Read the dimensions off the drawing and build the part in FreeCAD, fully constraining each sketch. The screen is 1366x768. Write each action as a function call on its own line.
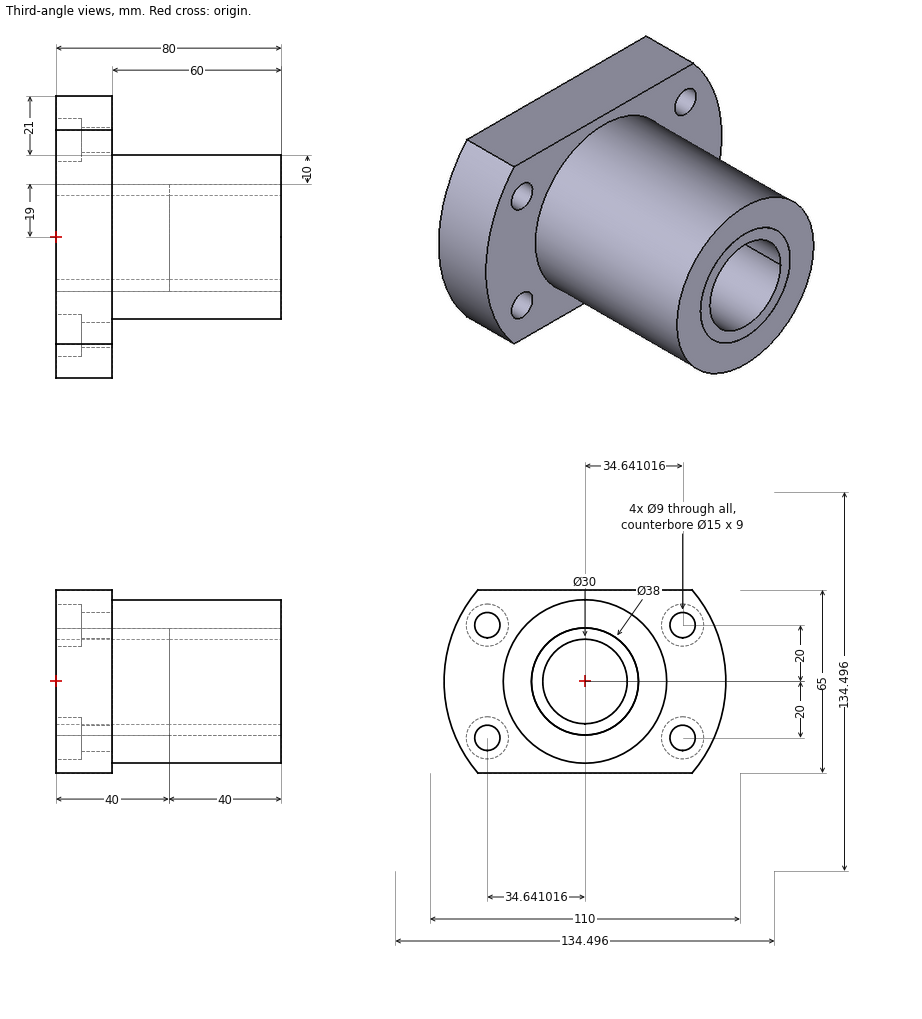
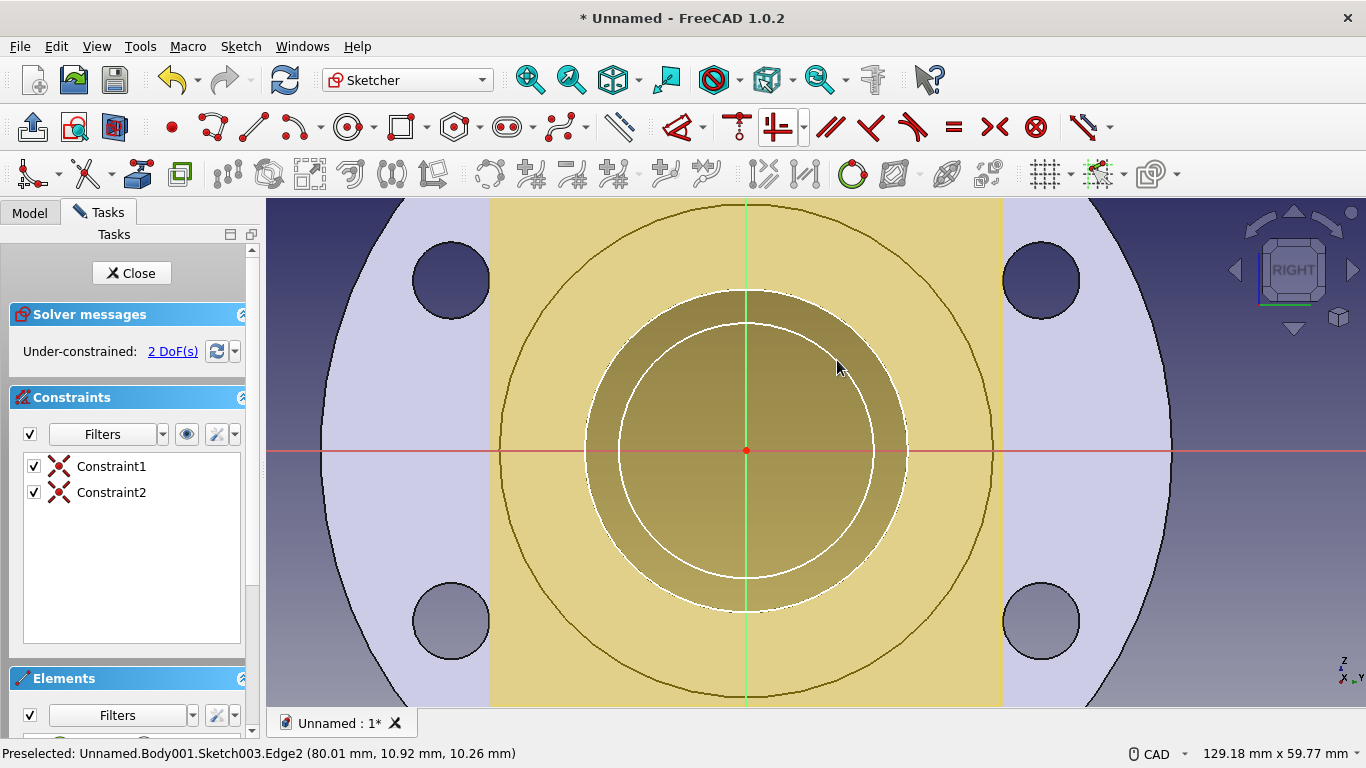
key(d)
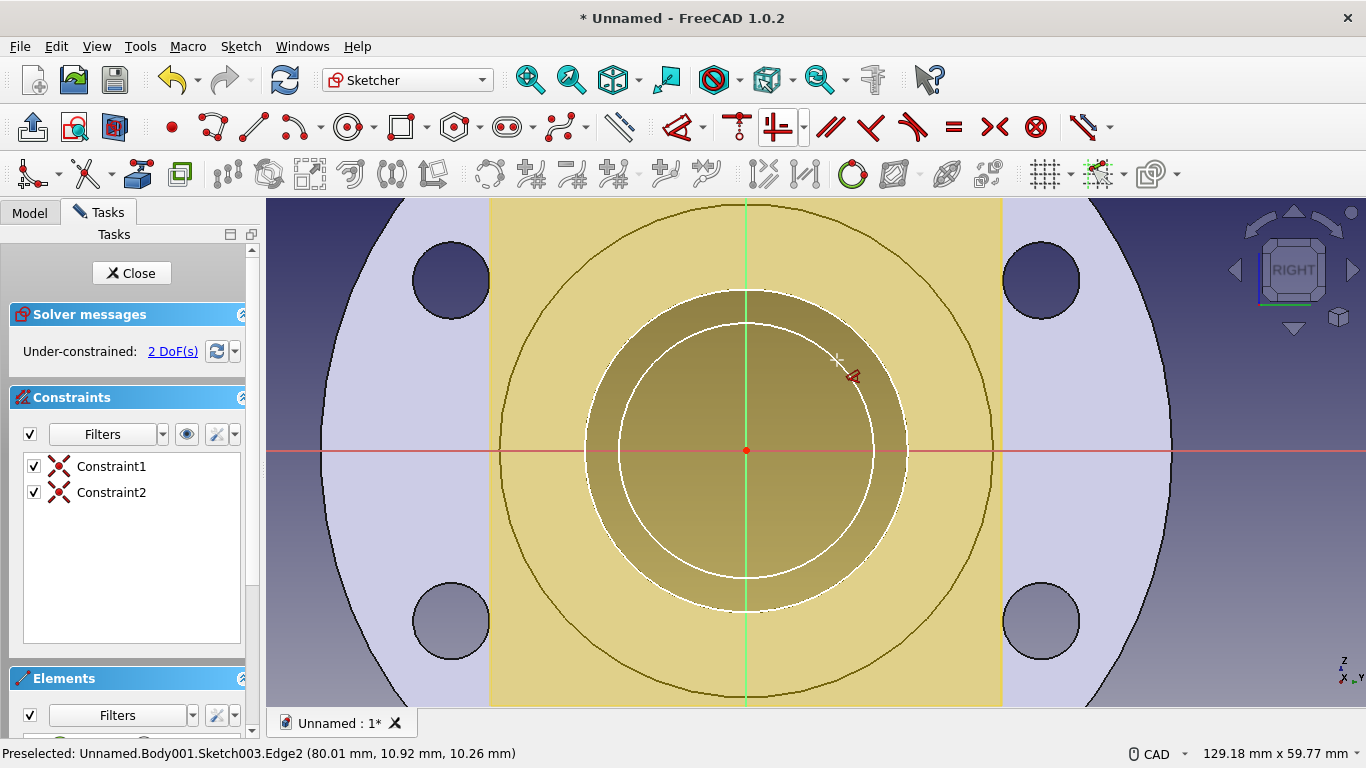
click(860, 336)
click(883, 313)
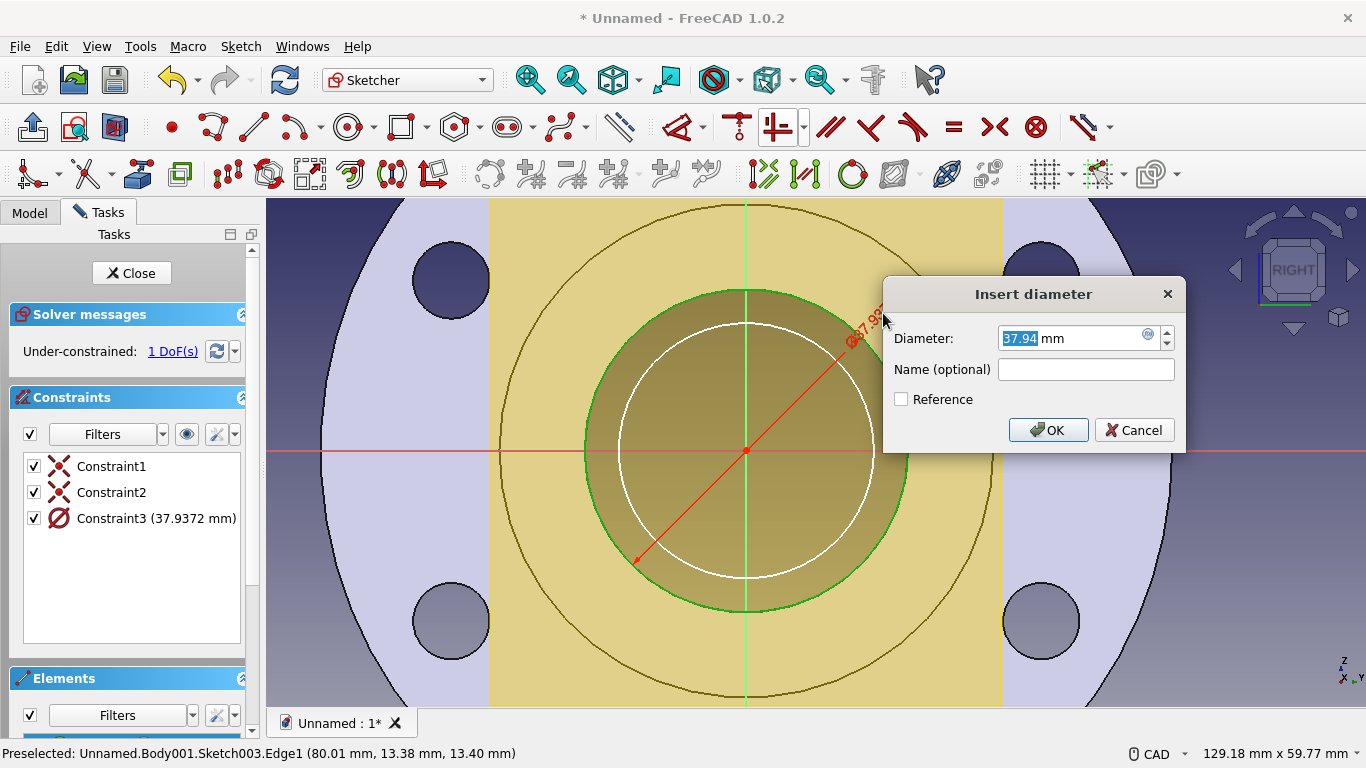
text(38)
key(Return)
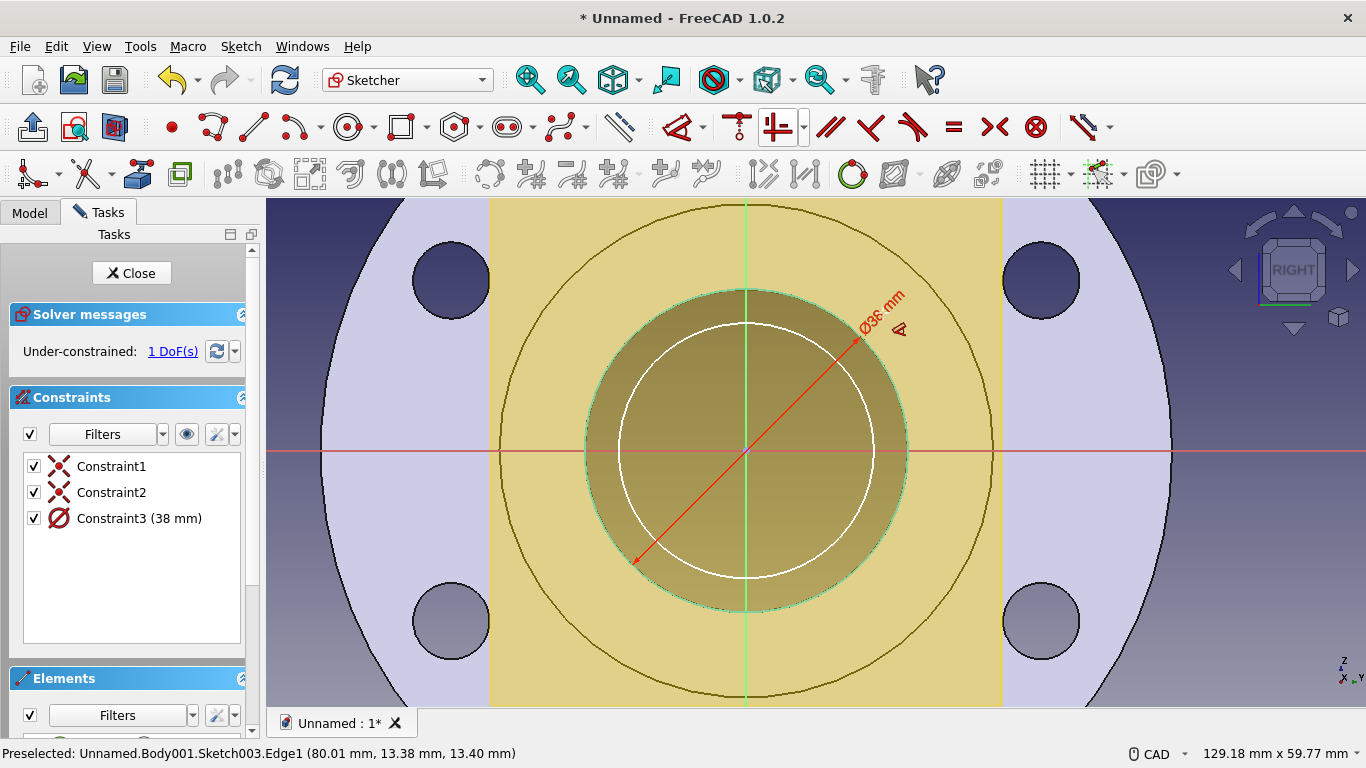
click(836, 360)
click(921, 398)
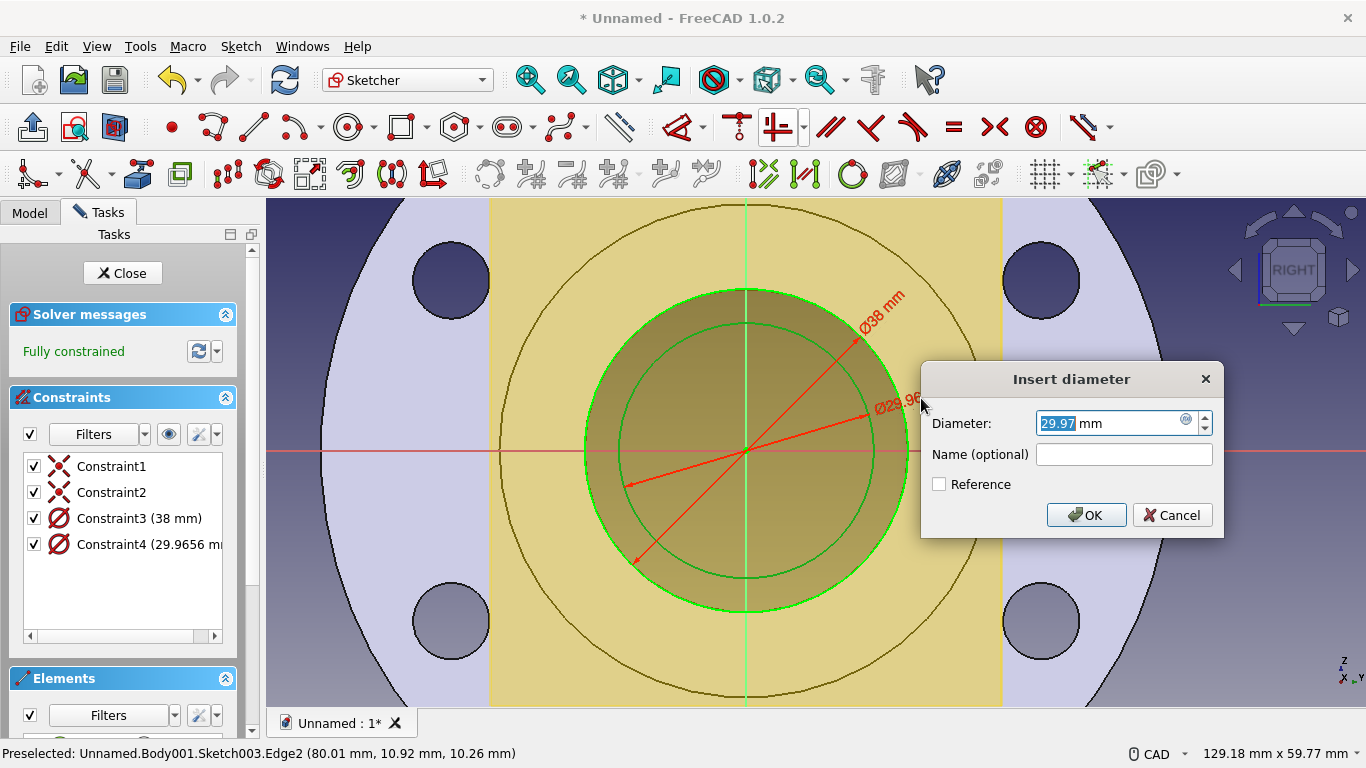
text(30)
key(Return)
key(Escape)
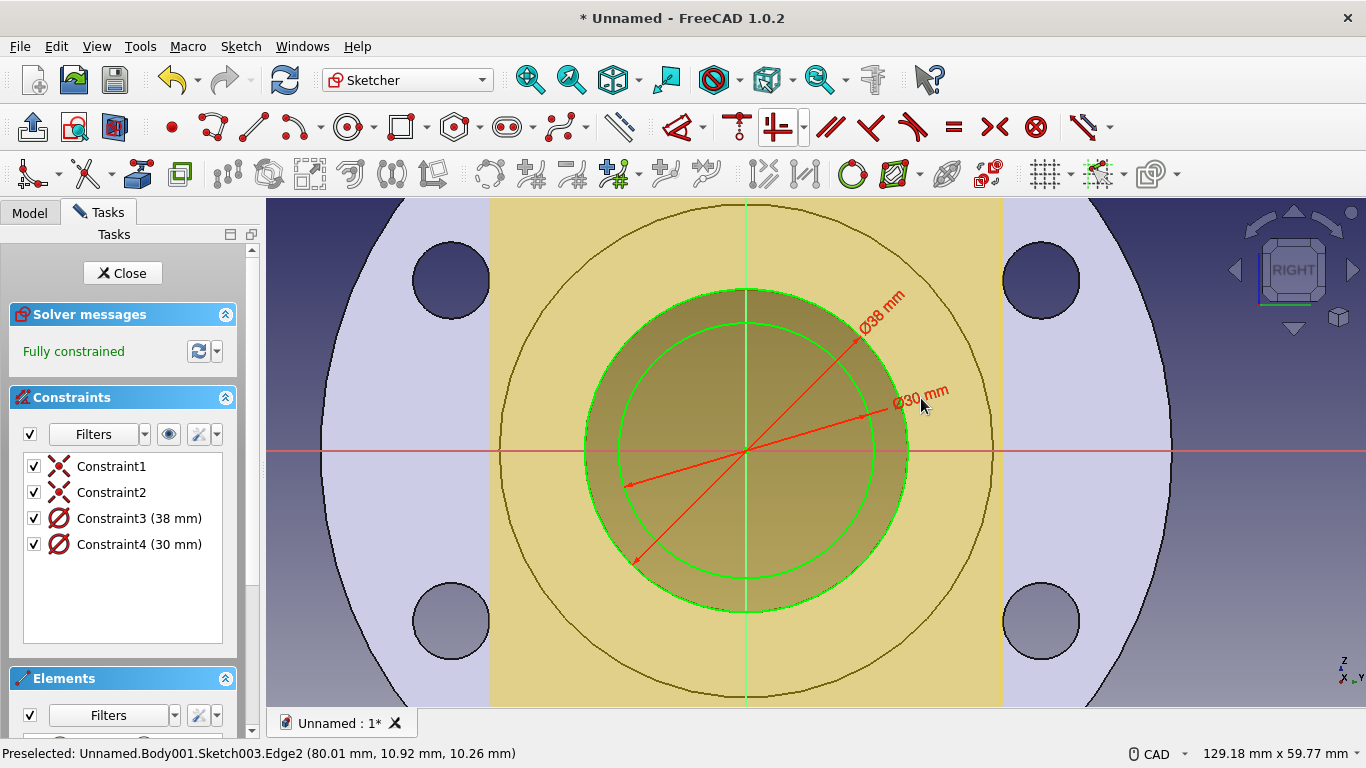
click(123, 273)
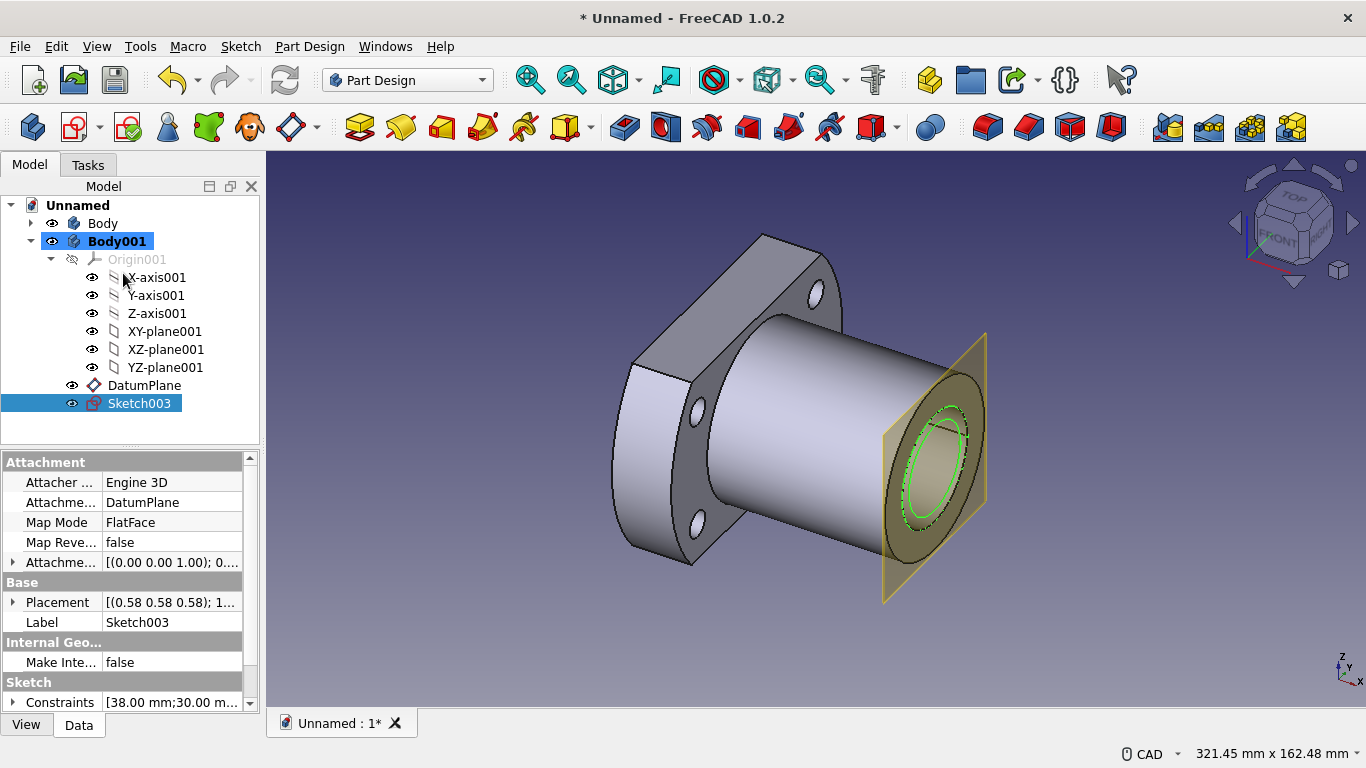
click(360, 128)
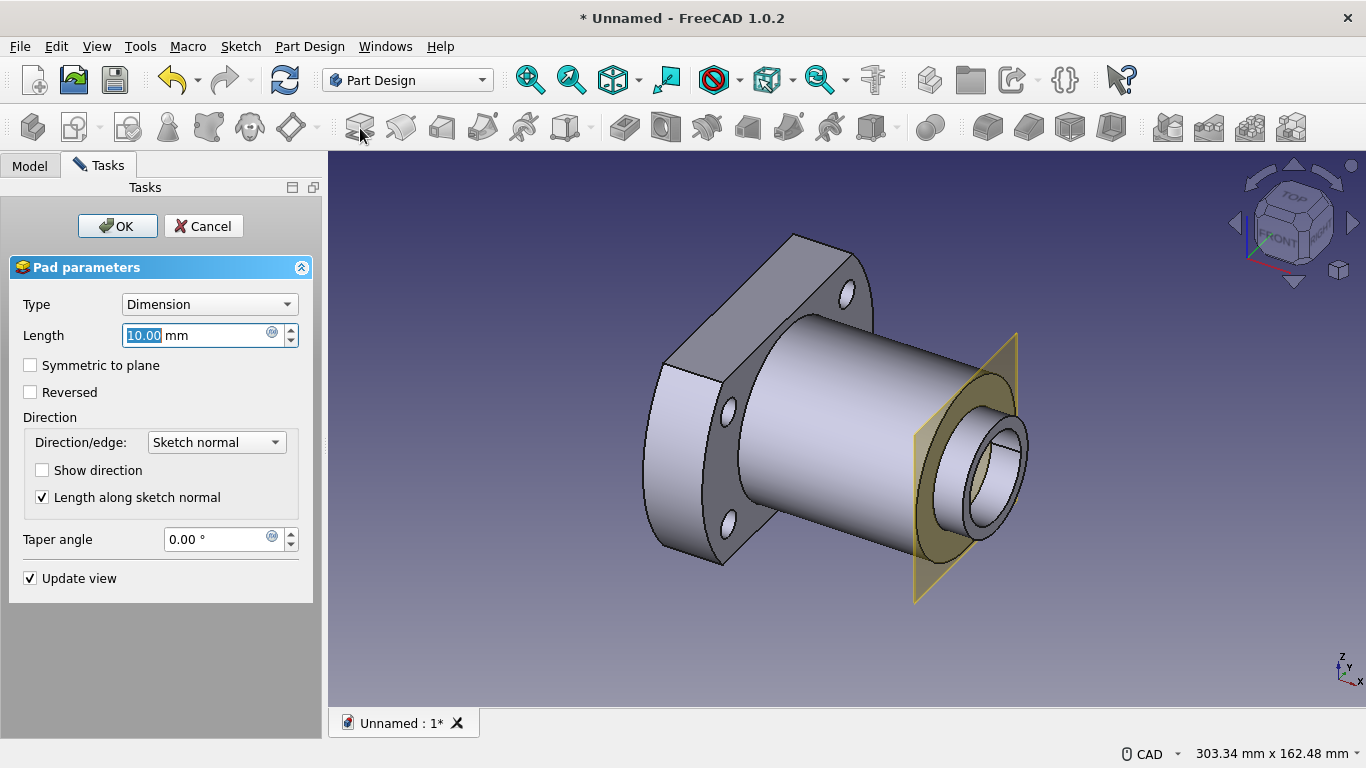
text(40)
key(Tab)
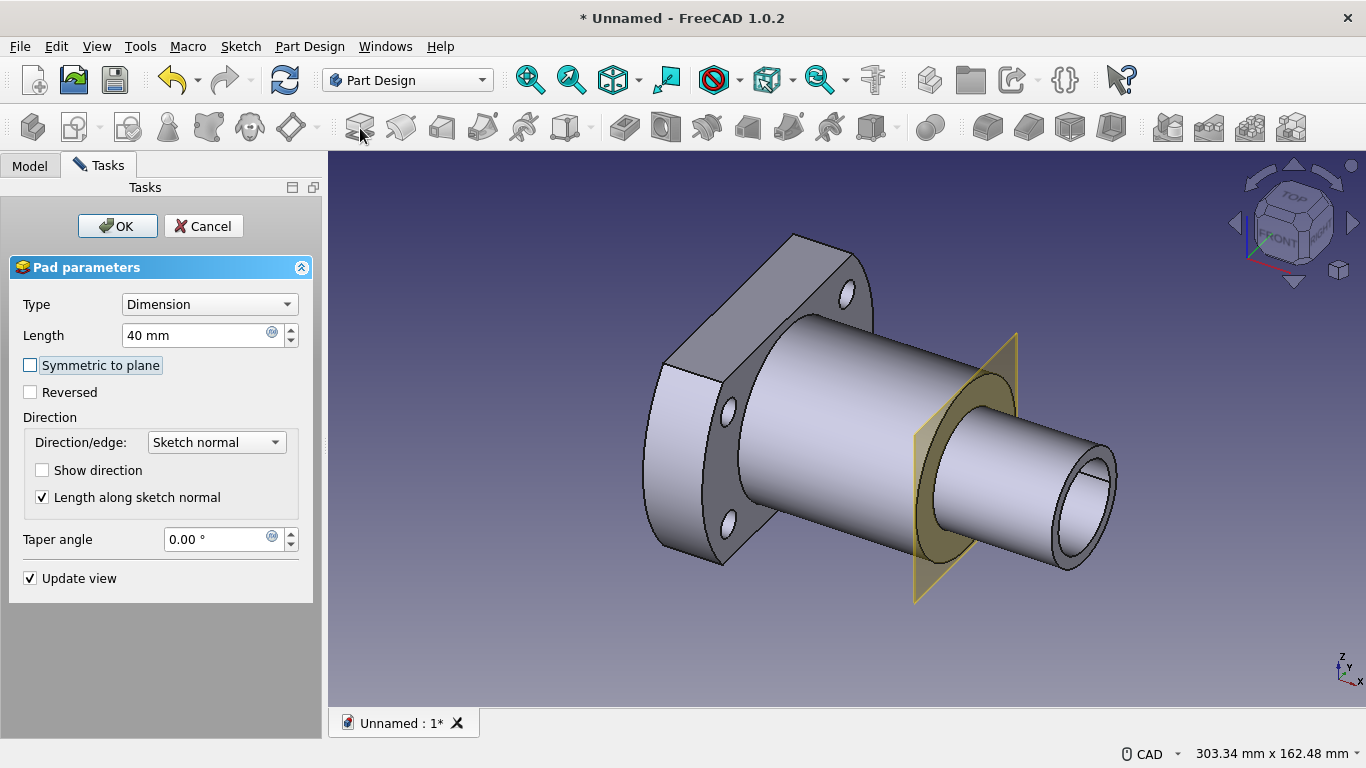
click(31, 392)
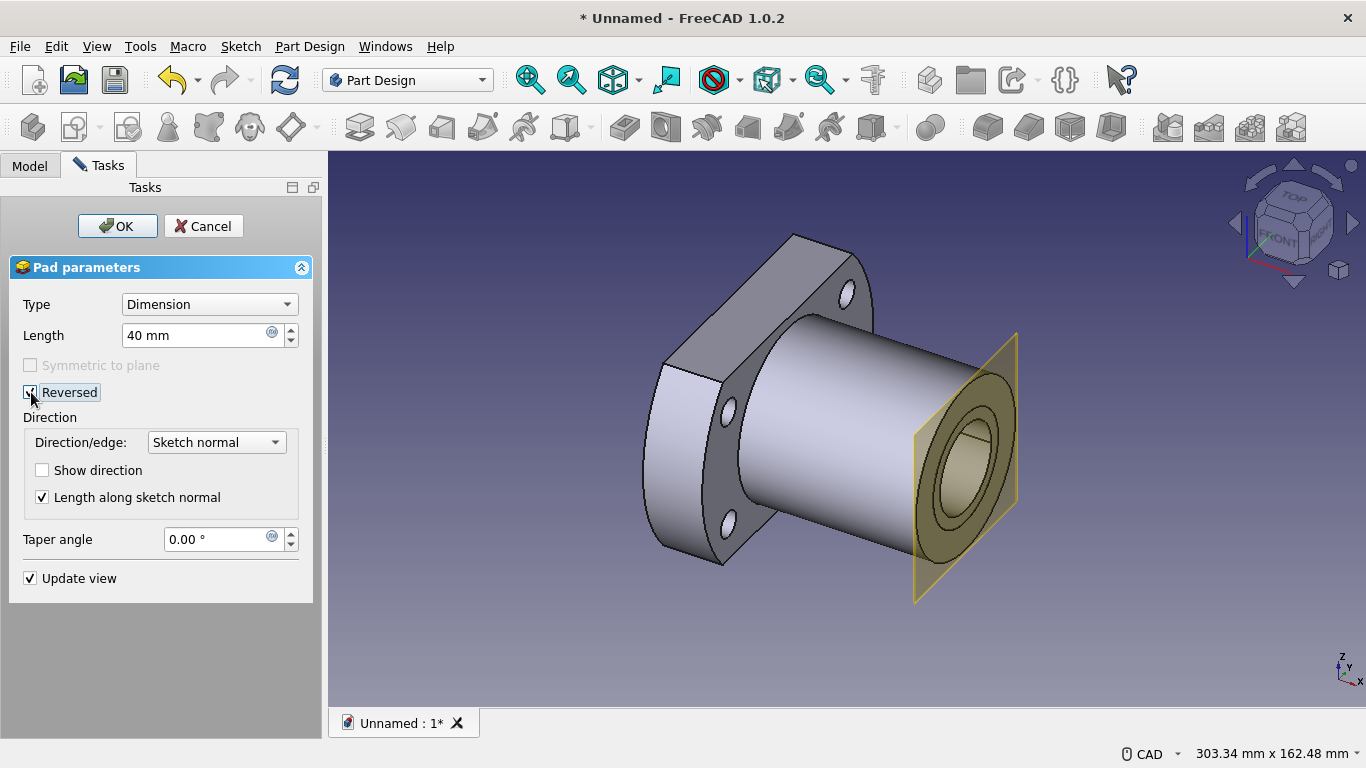
click(118, 226)